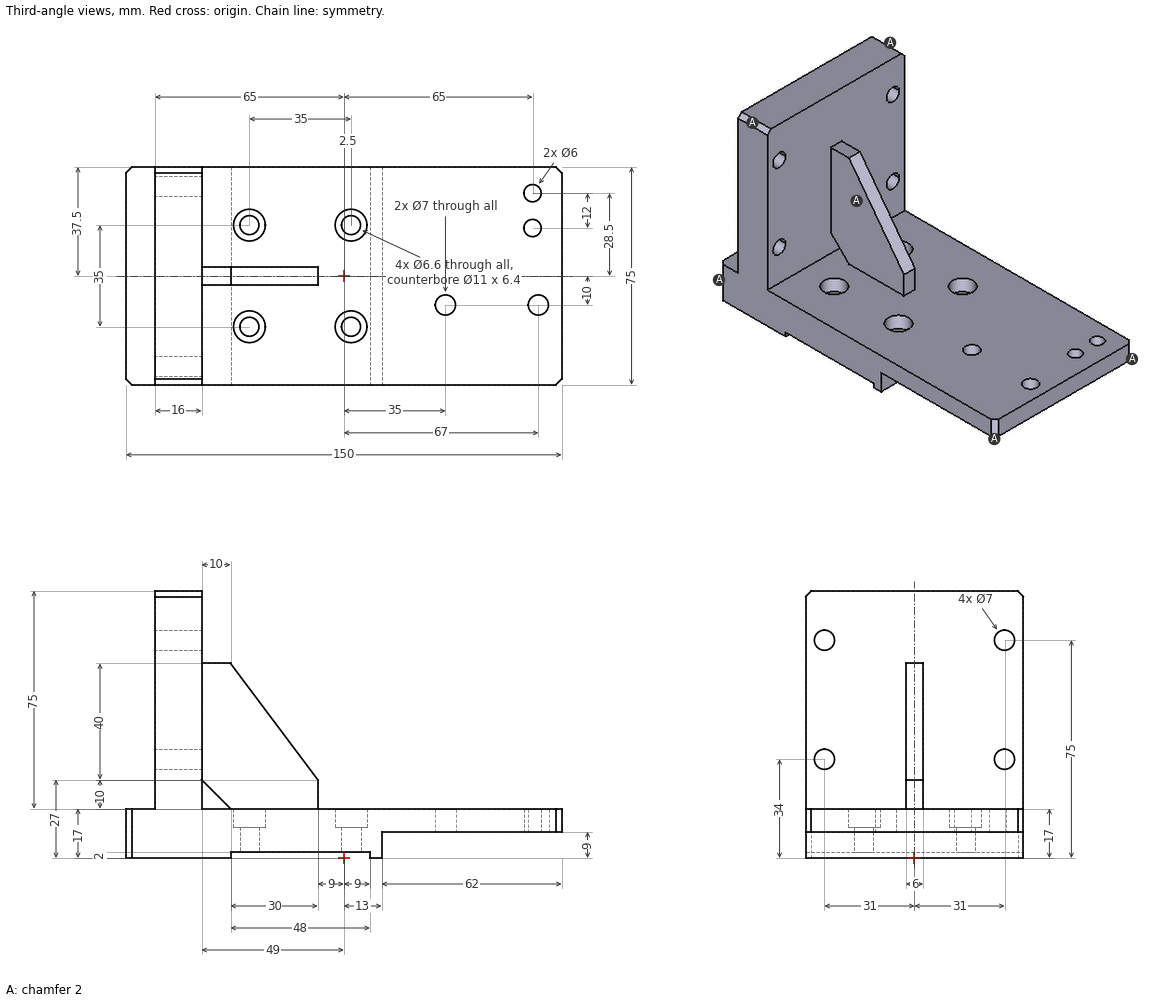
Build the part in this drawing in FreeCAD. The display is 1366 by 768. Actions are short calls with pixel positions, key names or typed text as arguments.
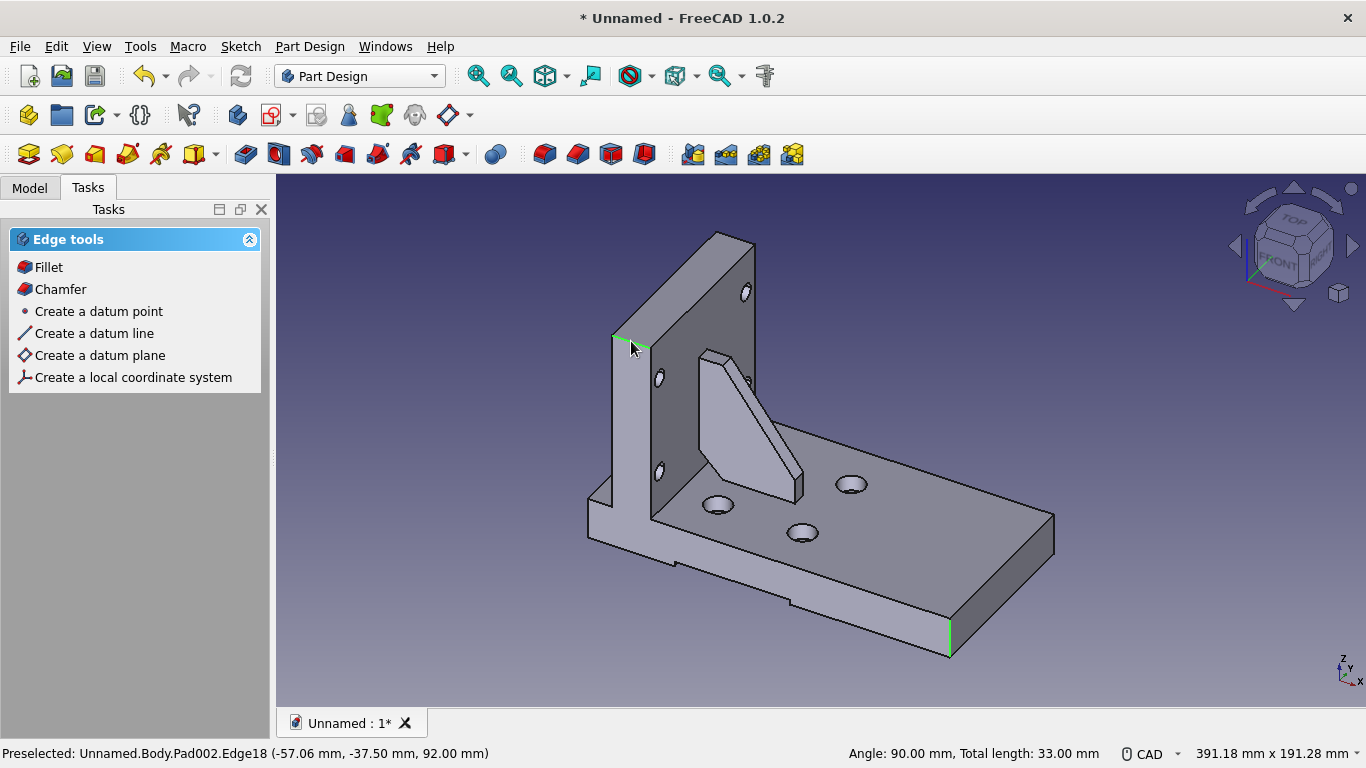
key(0)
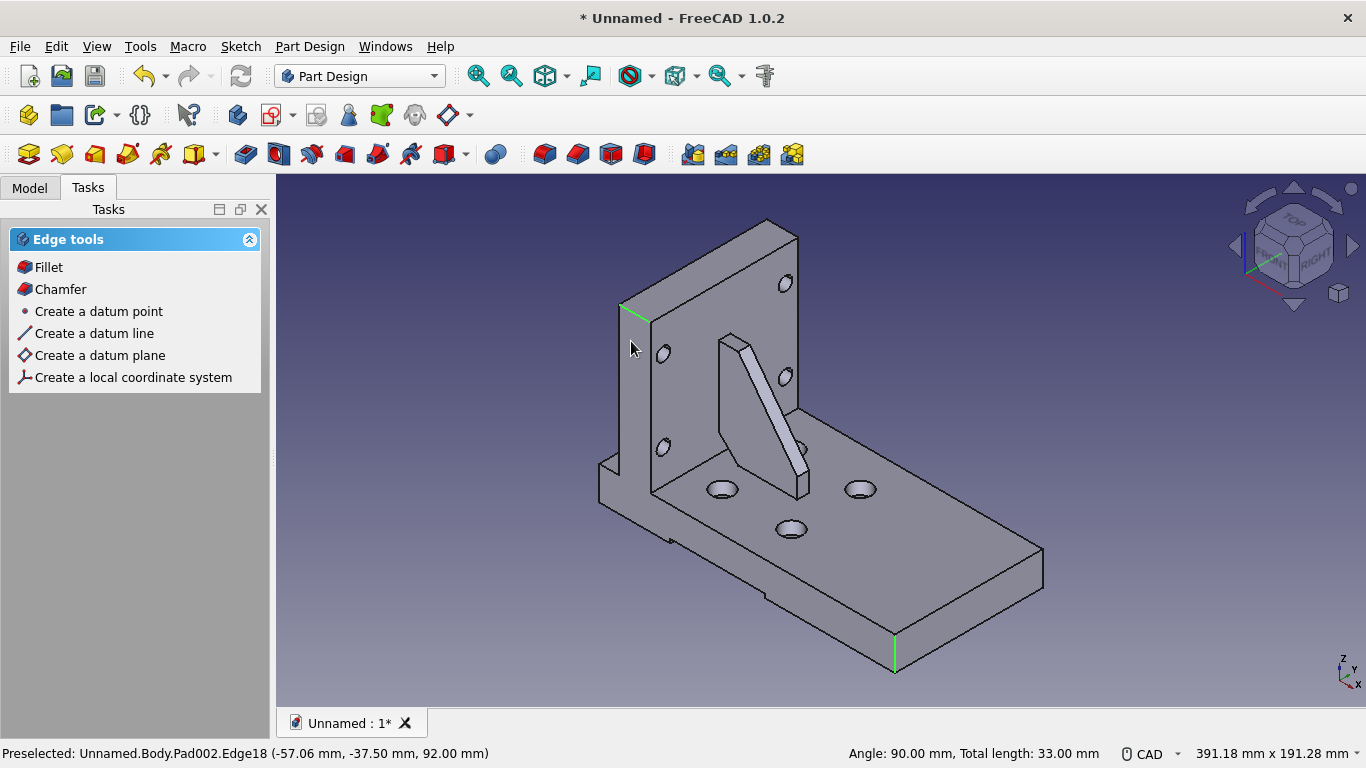
key(2)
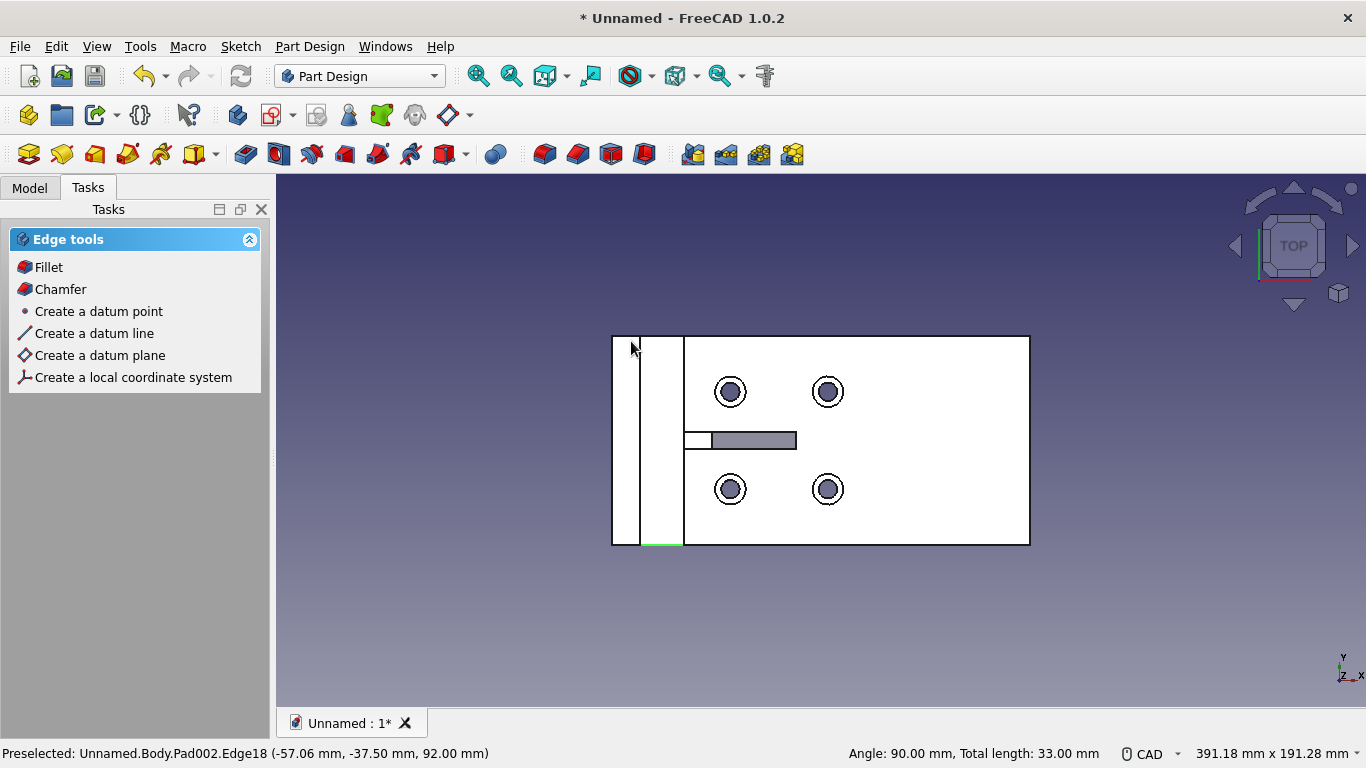
click(479, 76)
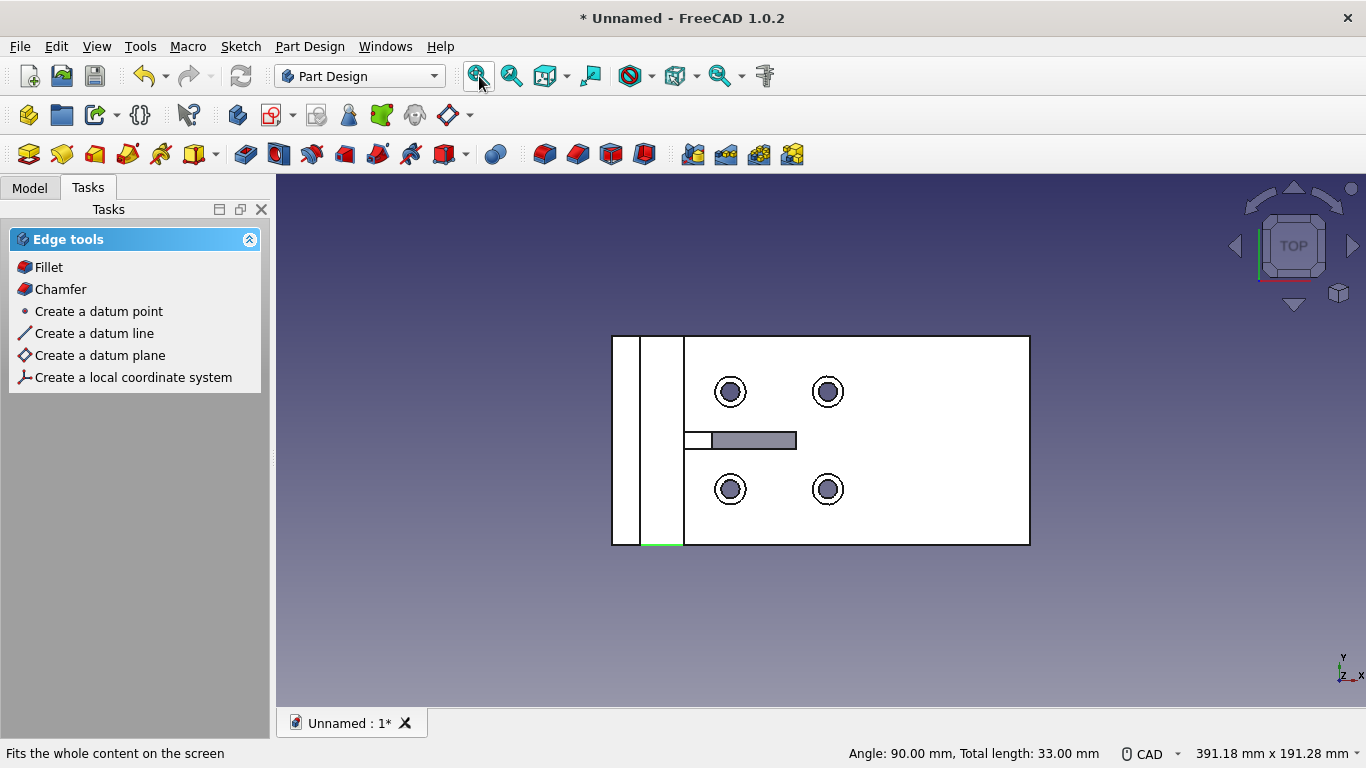
click(662, 335, ctrl)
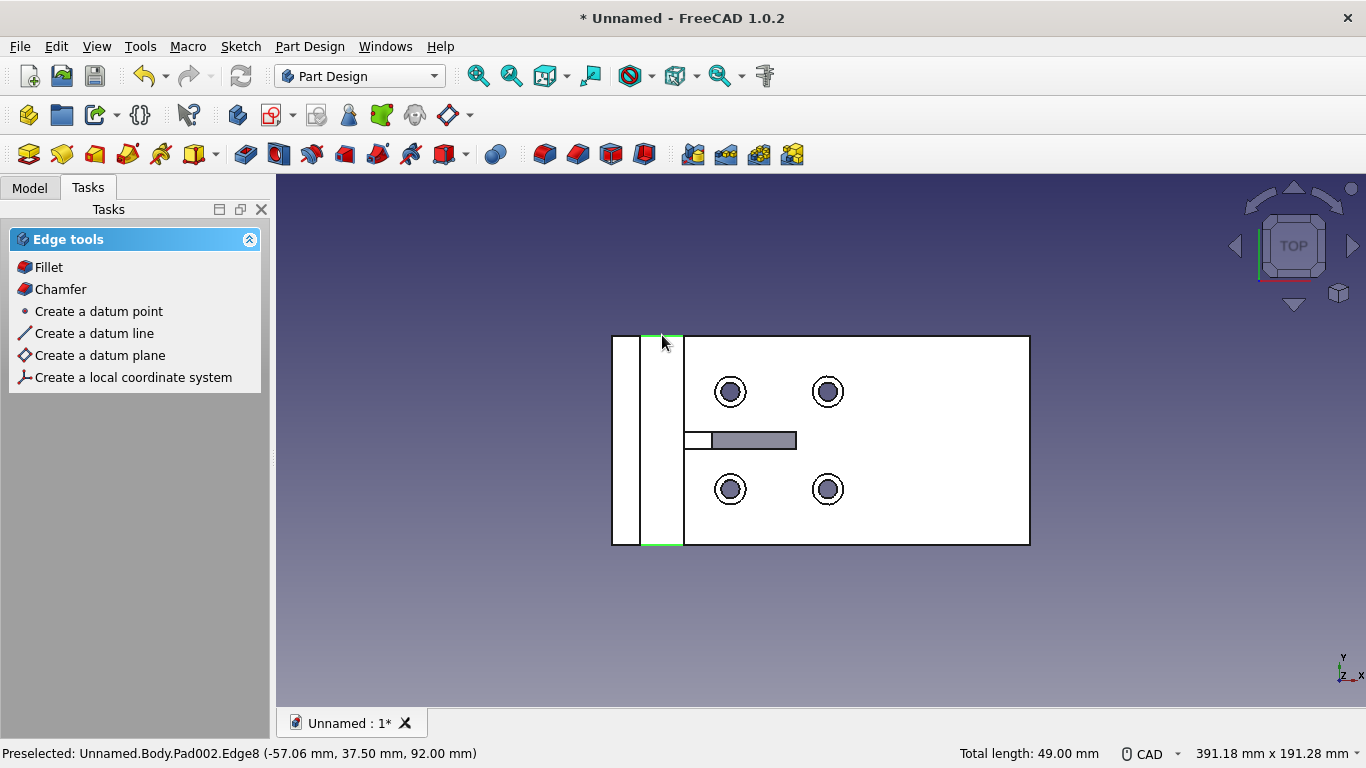
key(1)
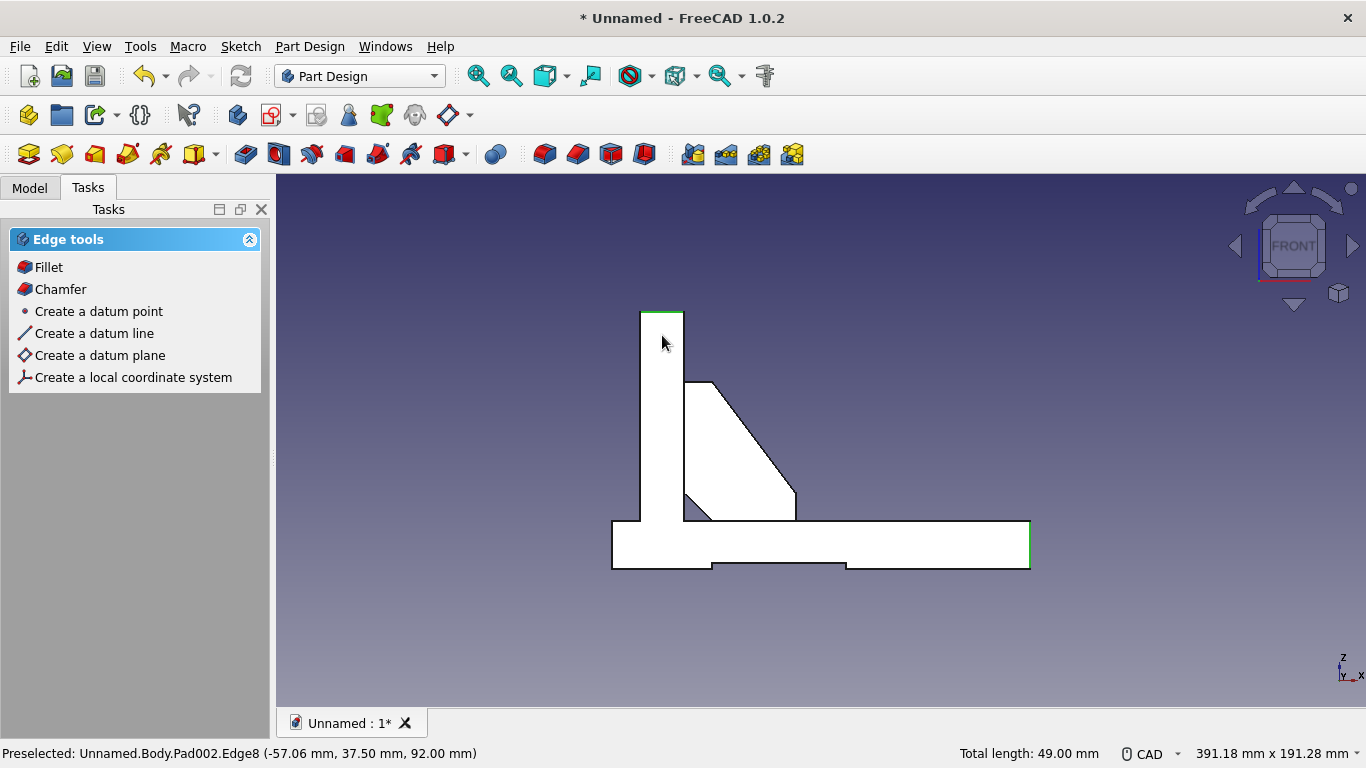
click(612, 544, ctrl)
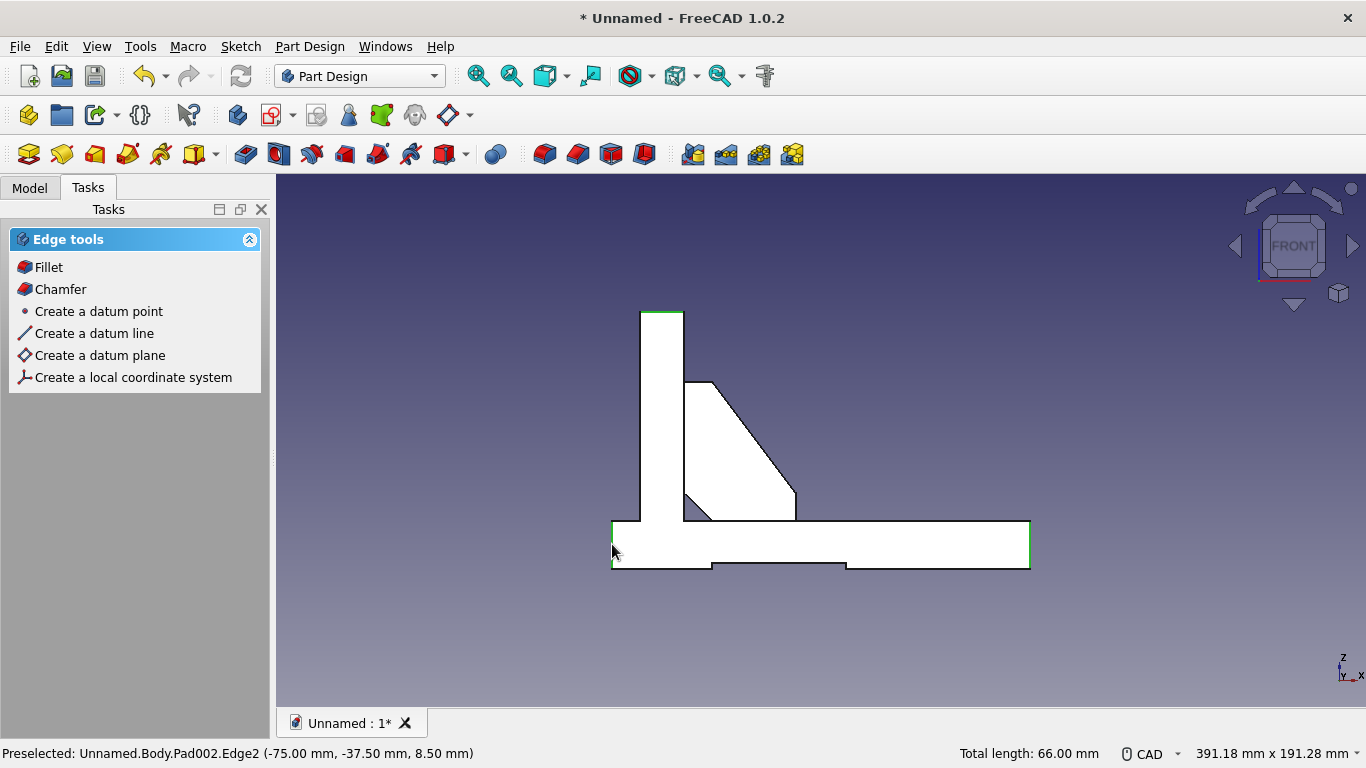
key(3)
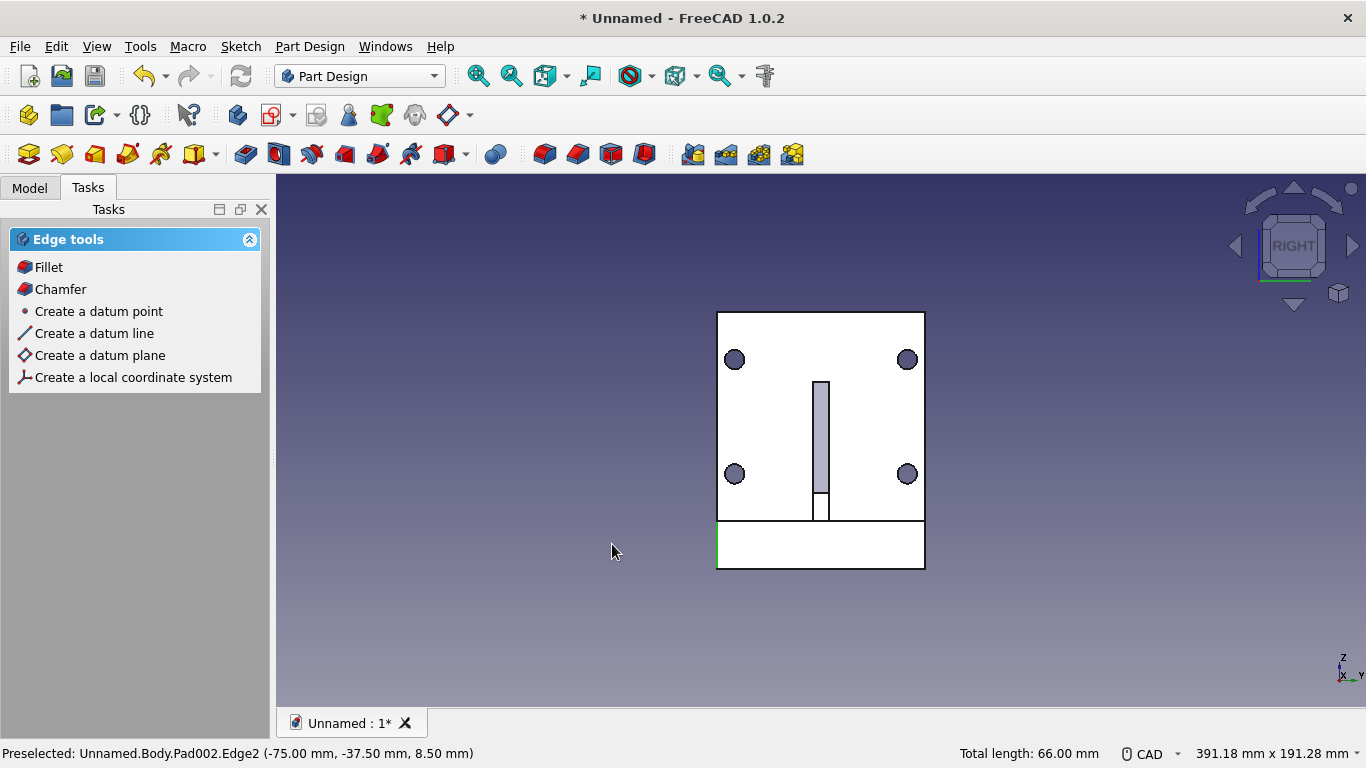
click(925, 544, ctrl)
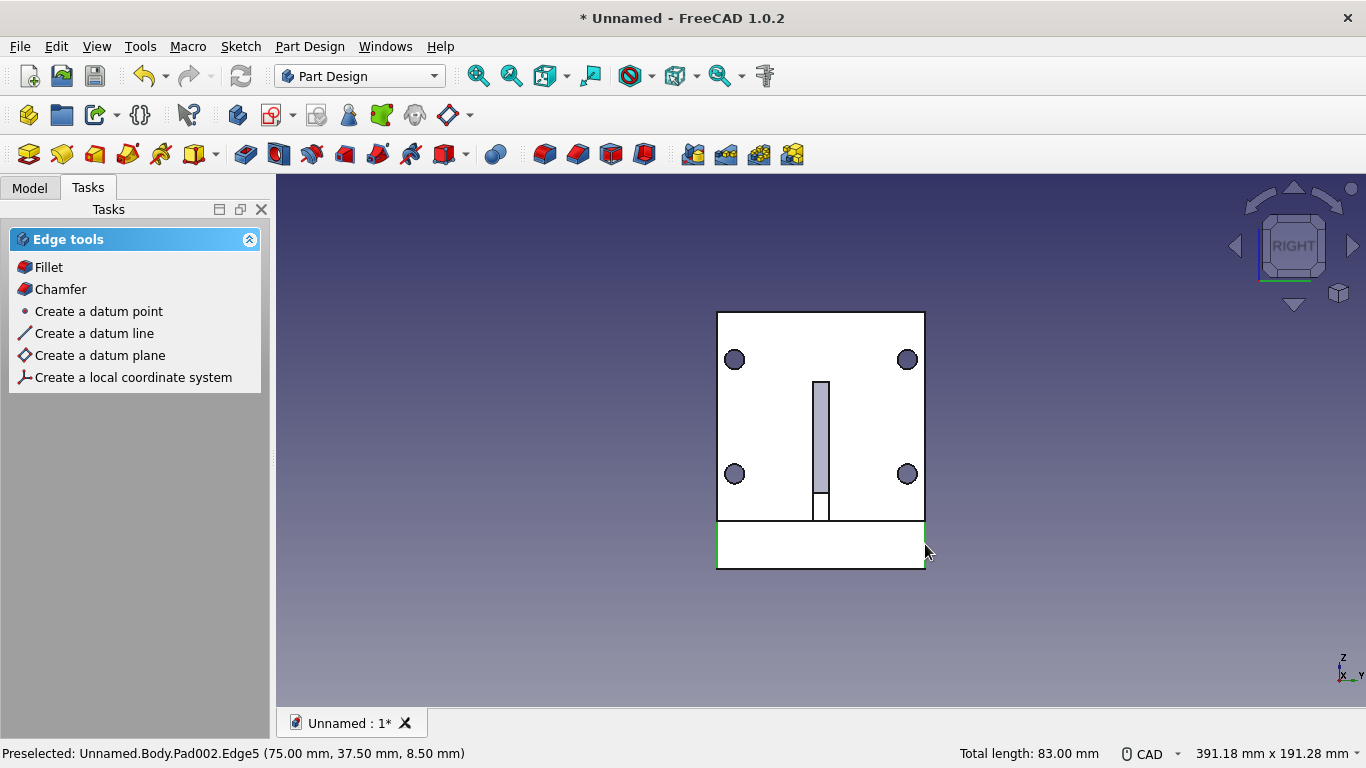
key(5)